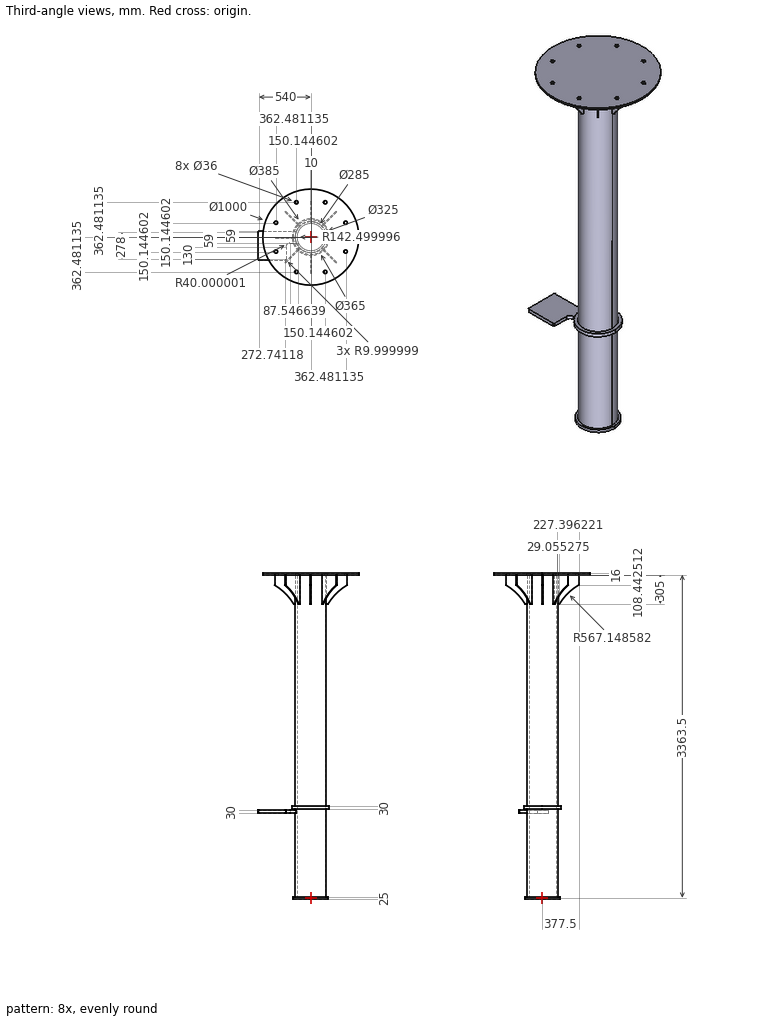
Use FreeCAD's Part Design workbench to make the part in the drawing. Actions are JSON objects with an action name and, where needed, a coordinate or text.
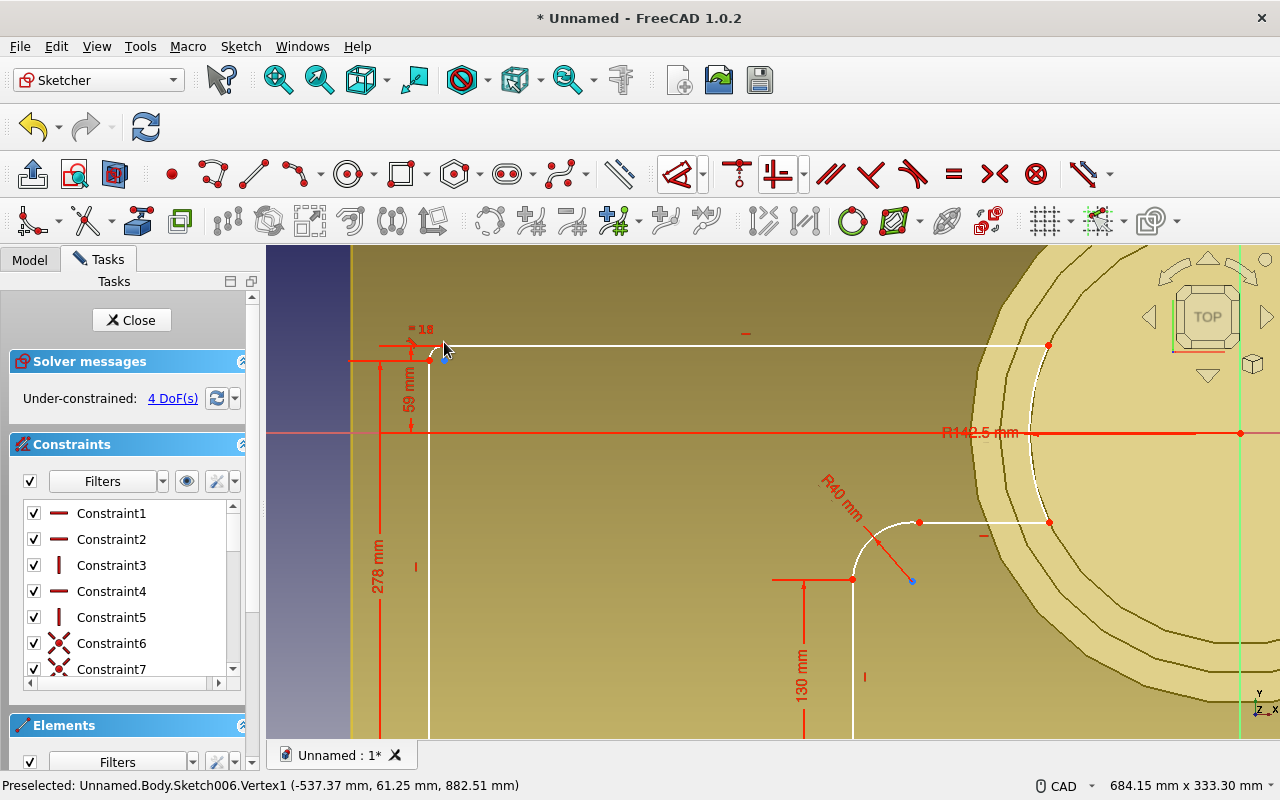
{"action": "scroll", "coordinate": [1049, 523], "scroll_direction": "up", "scroll_amount": 12}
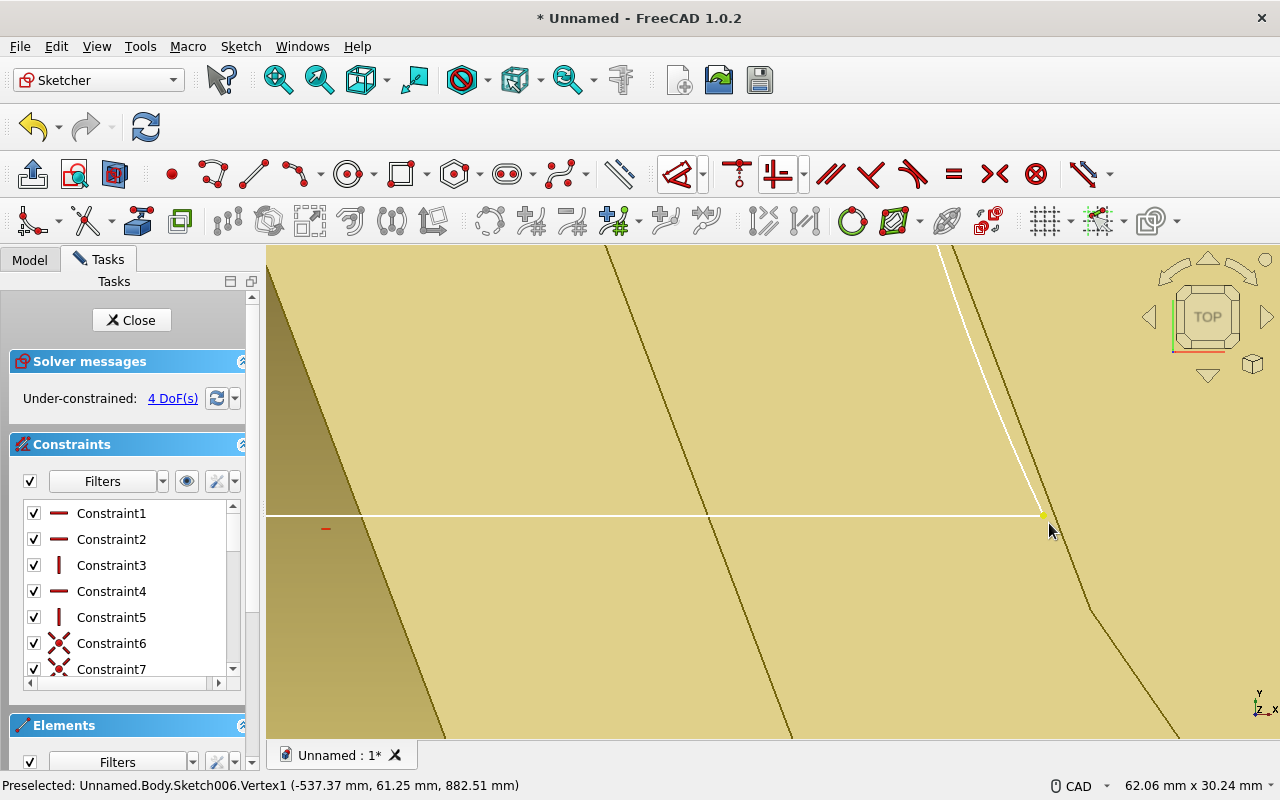
{"action": "left_click", "coordinate": [1044, 516]}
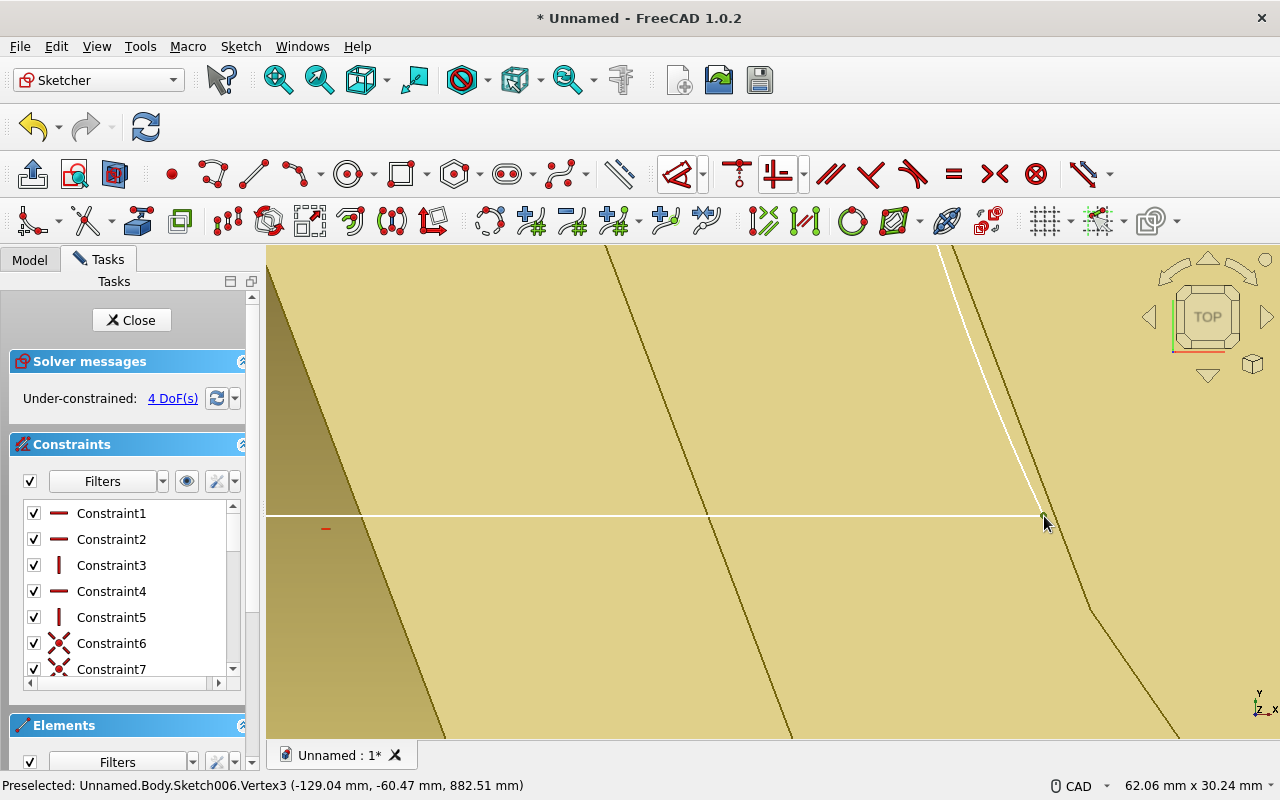
{"action": "key", "text": "i"}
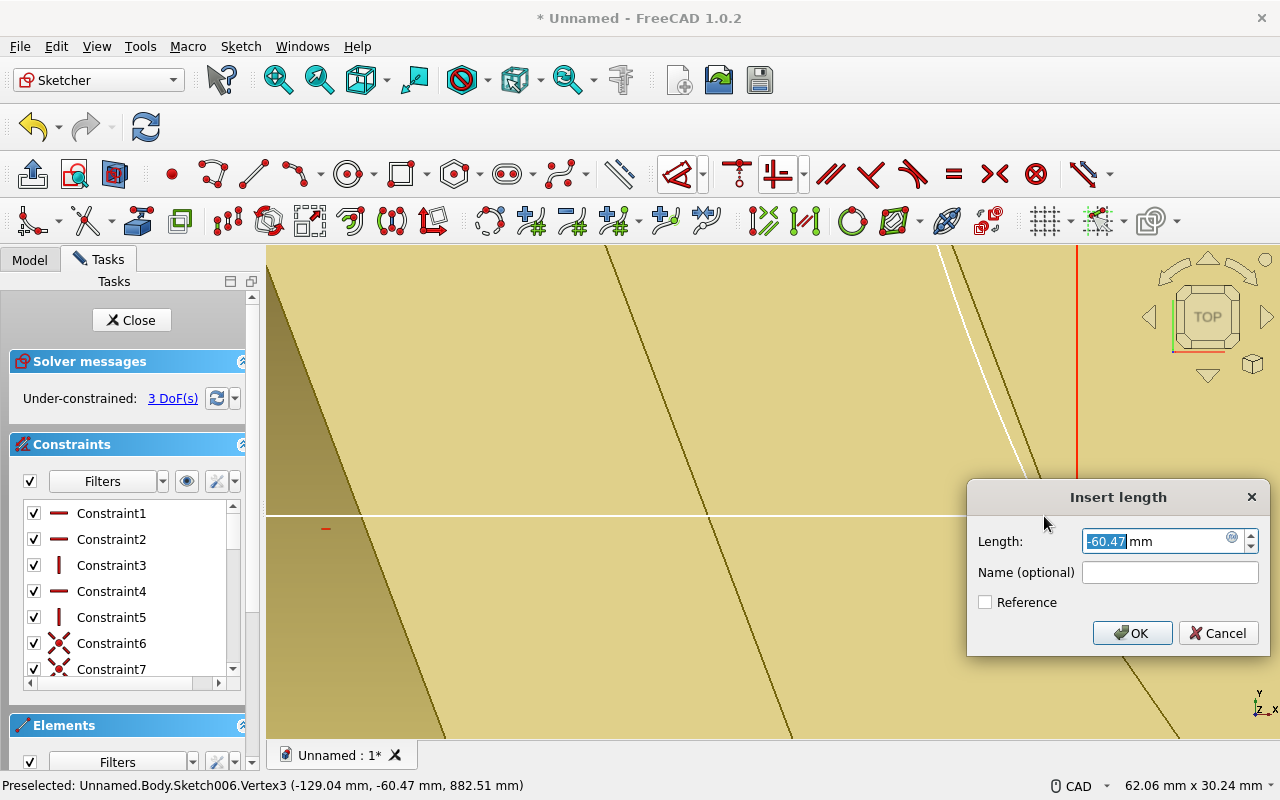
{"action": "type", "text": "-59"}
{"action": "key", "text": "Return"}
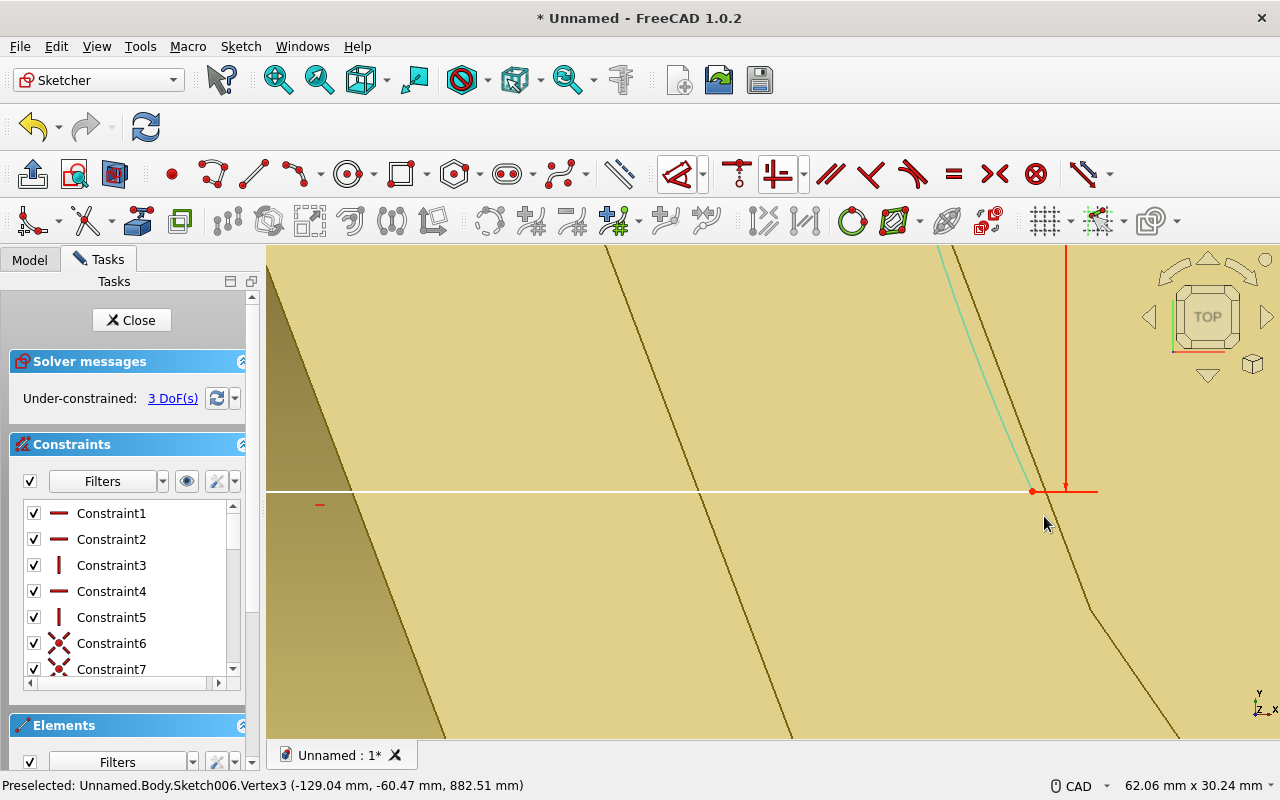
{"action": "scroll", "coordinate": [837, 459], "scroll_direction": "down", "scroll_amount": 14}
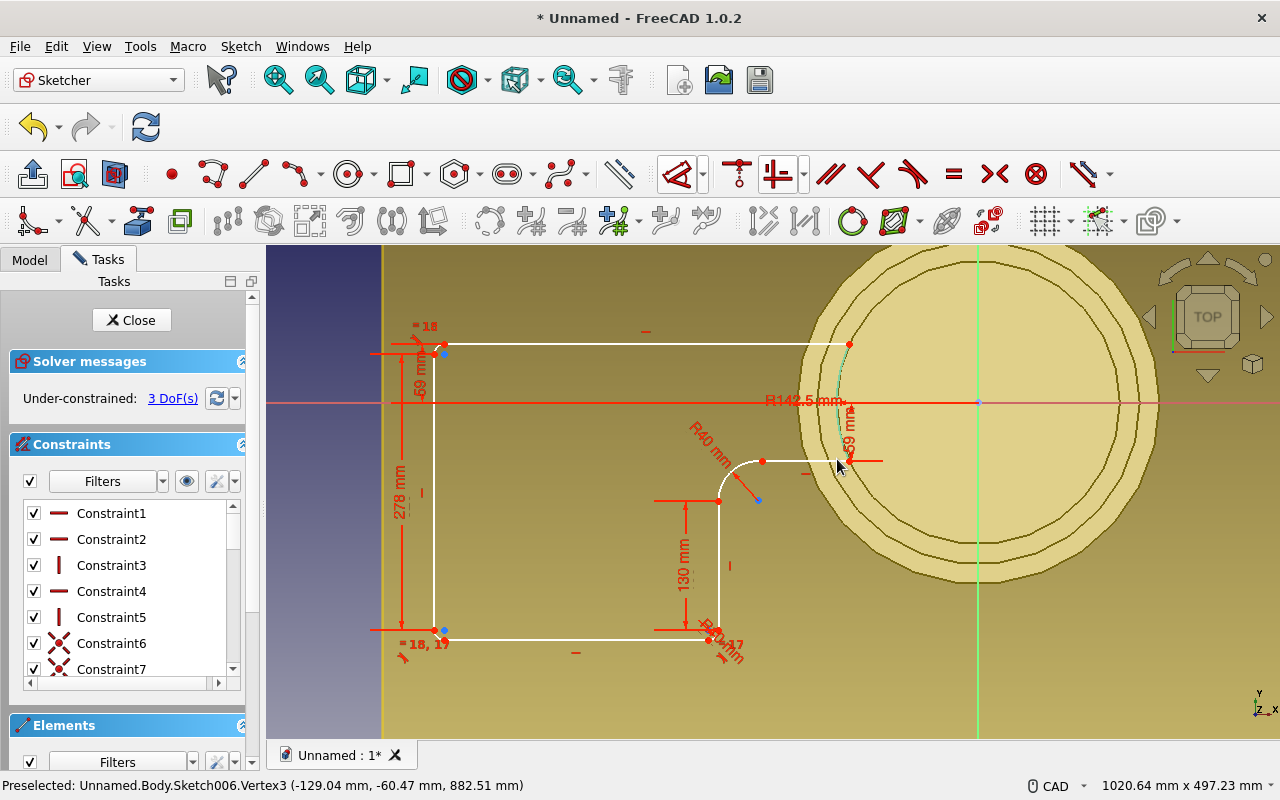
{"action": "scroll", "coordinate": [444, 344], "scroll_direction": "up", "scroll_amount": 2}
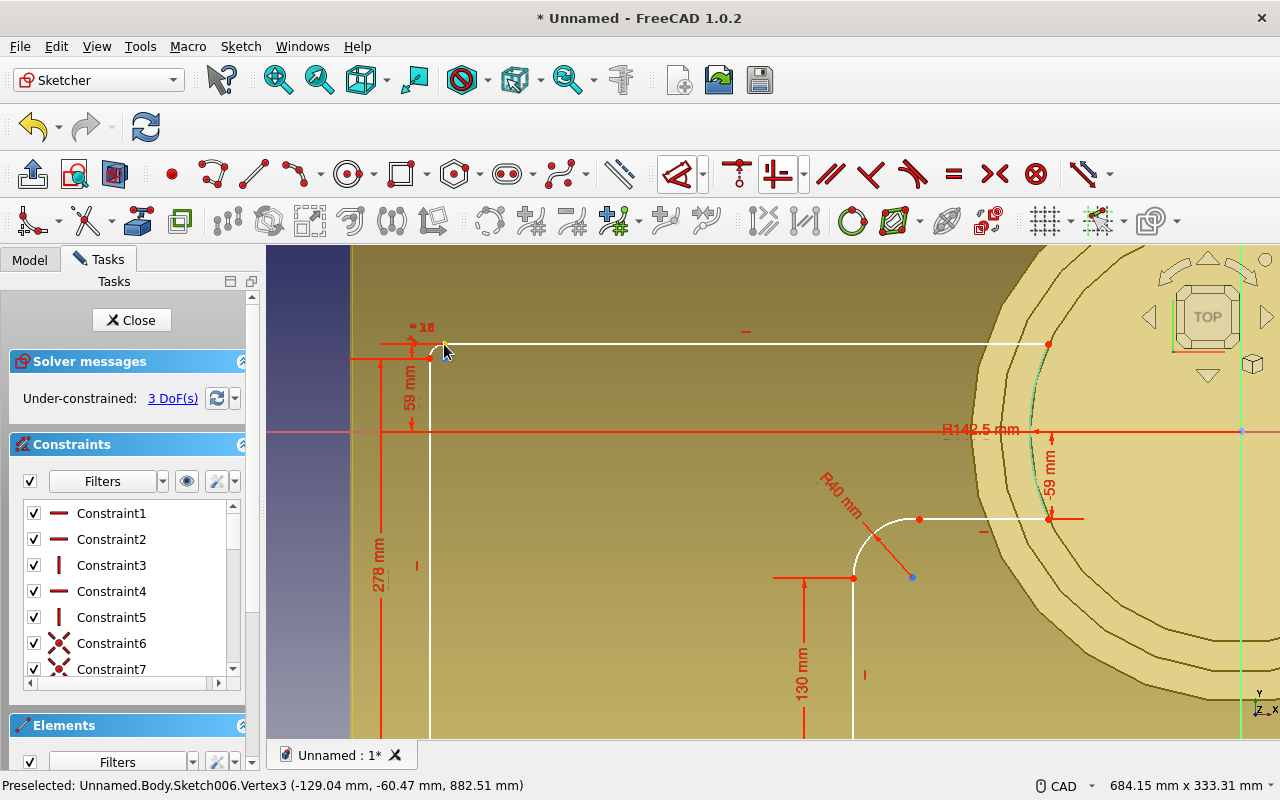
{"action": "left_click", "coordinate": [445, 344]}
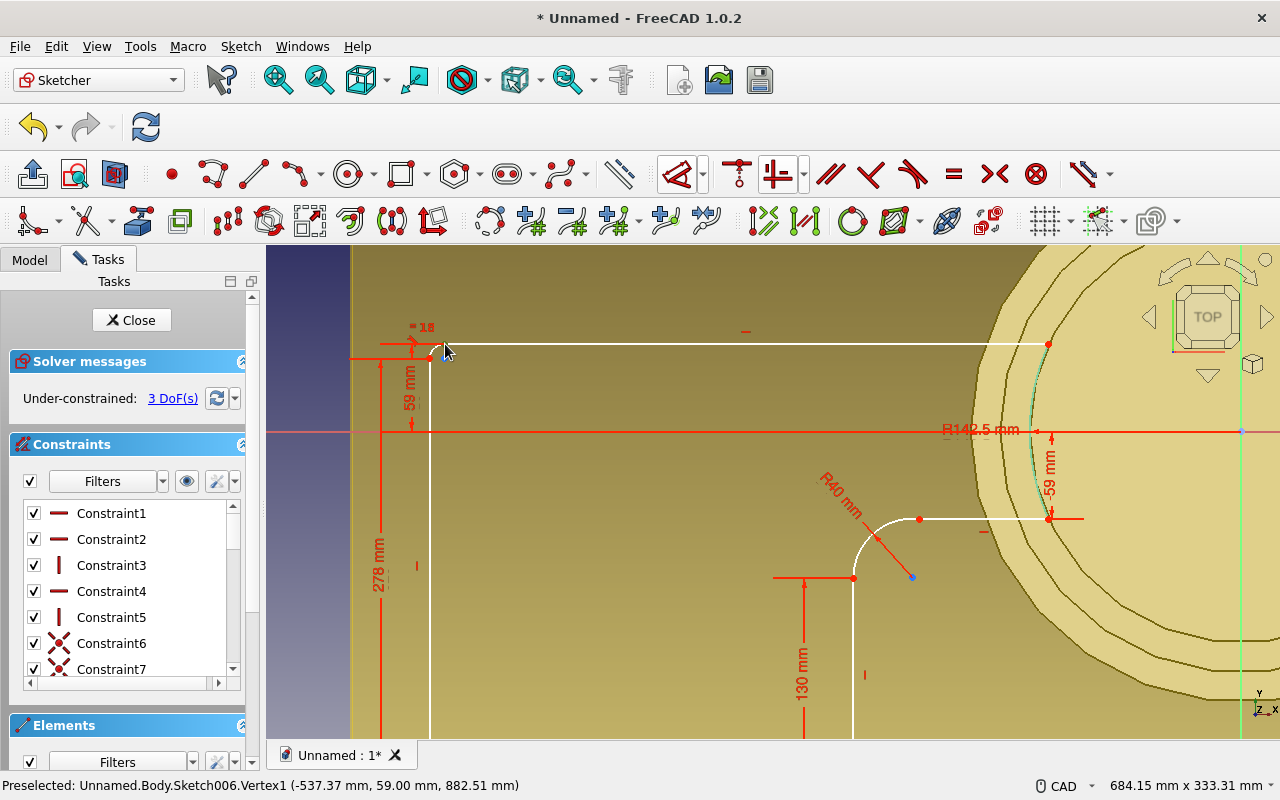
{"action": "key", "text": "l"}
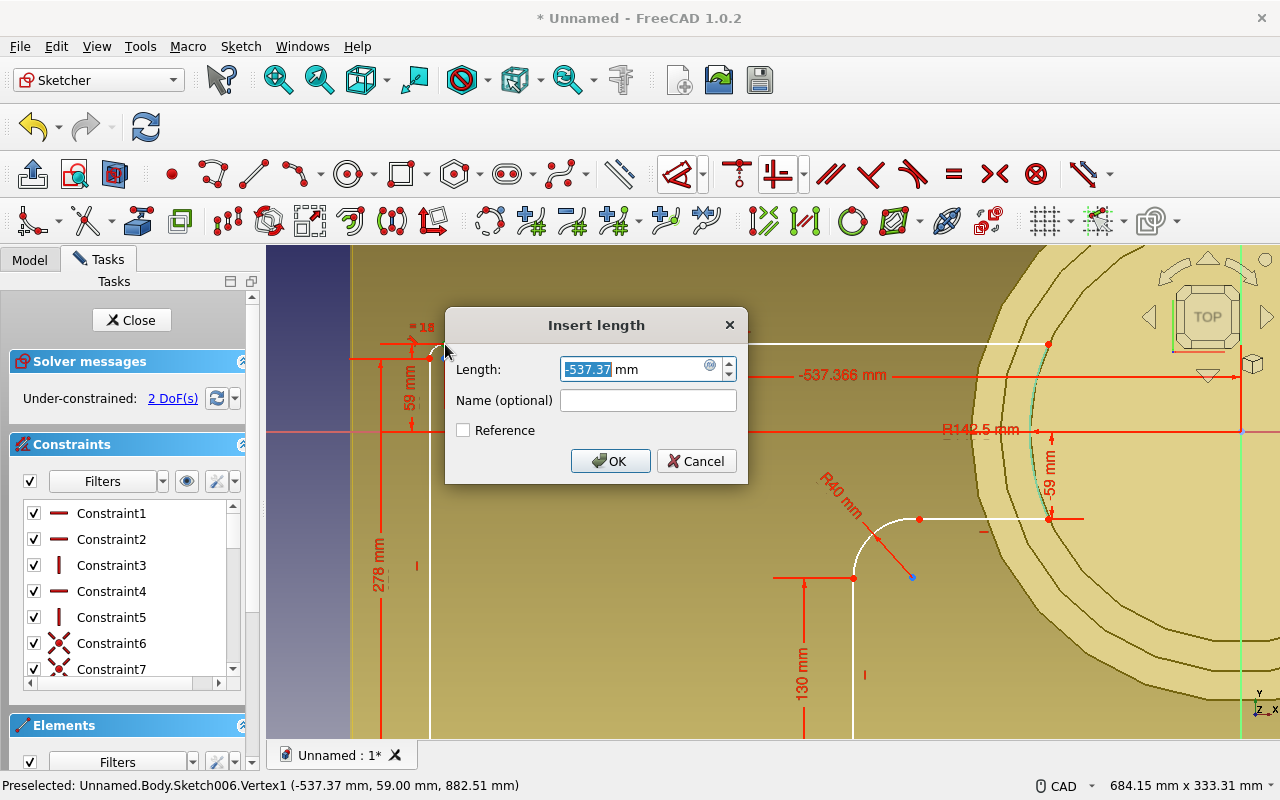
{"action": "type", "text": "-540"}
{"action": "key", "text": "Return"}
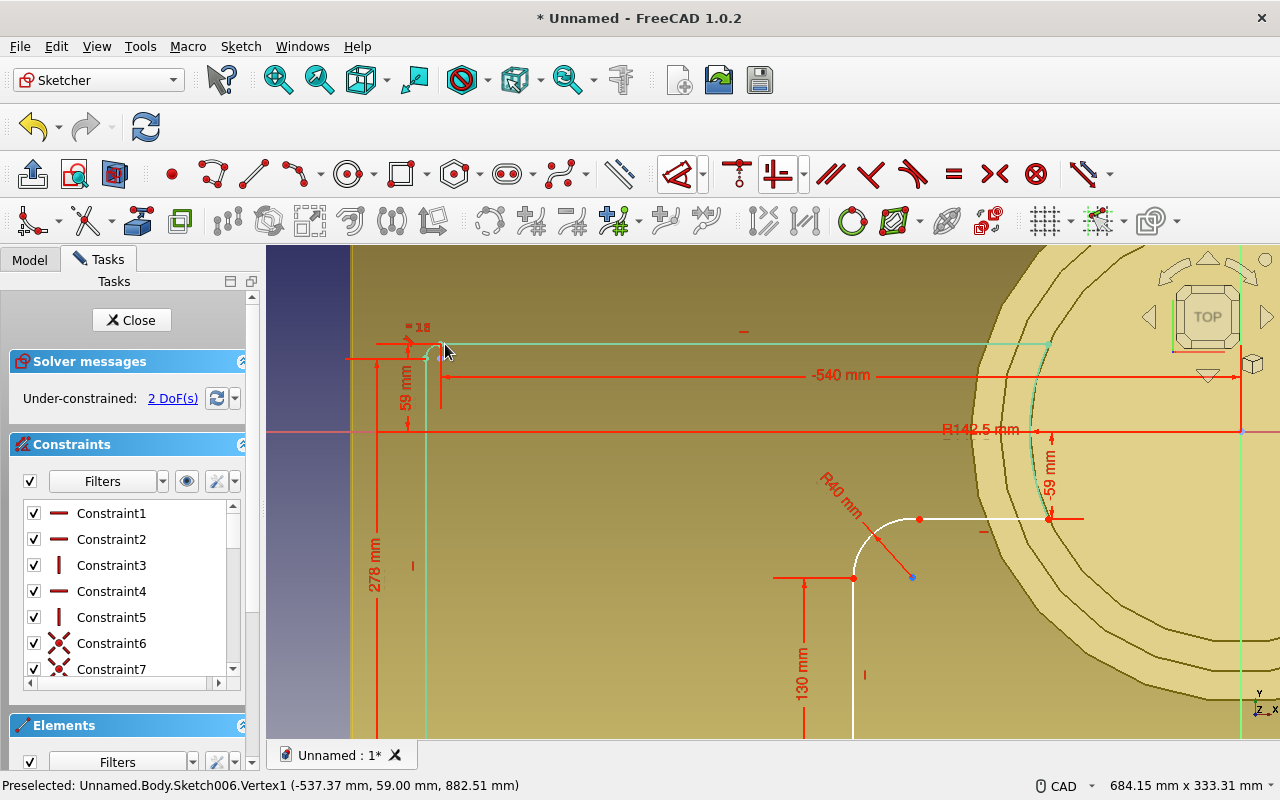
{"action": "left_click", "coordinate": [1010, 519]}